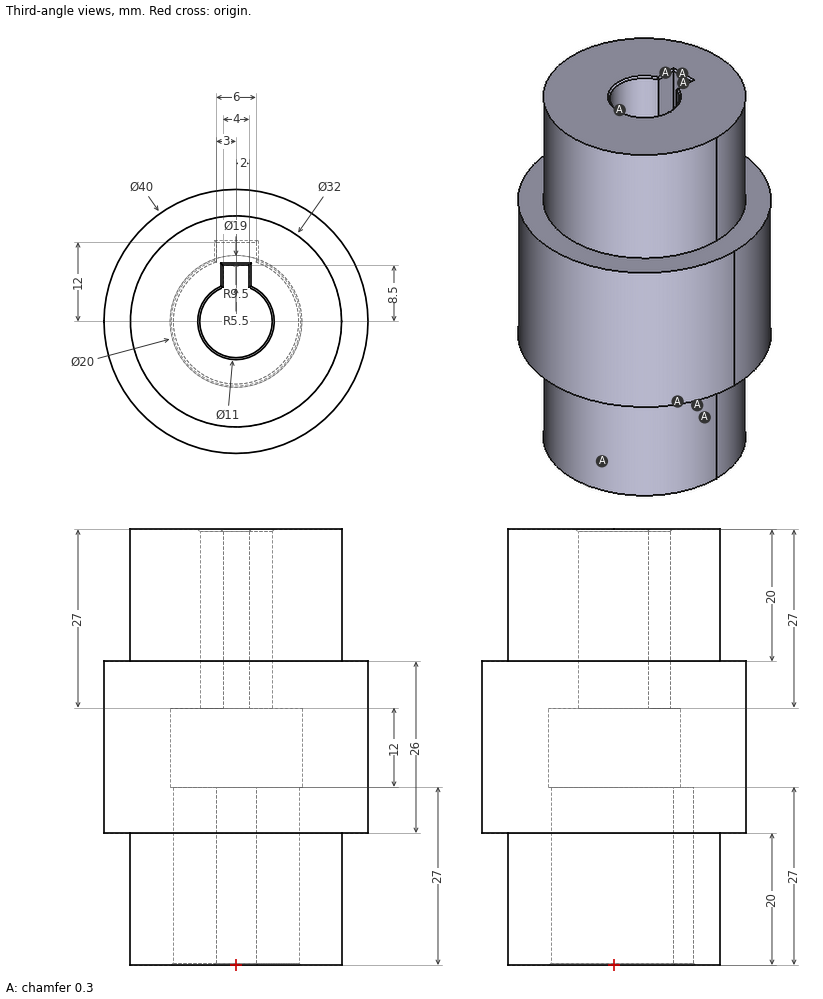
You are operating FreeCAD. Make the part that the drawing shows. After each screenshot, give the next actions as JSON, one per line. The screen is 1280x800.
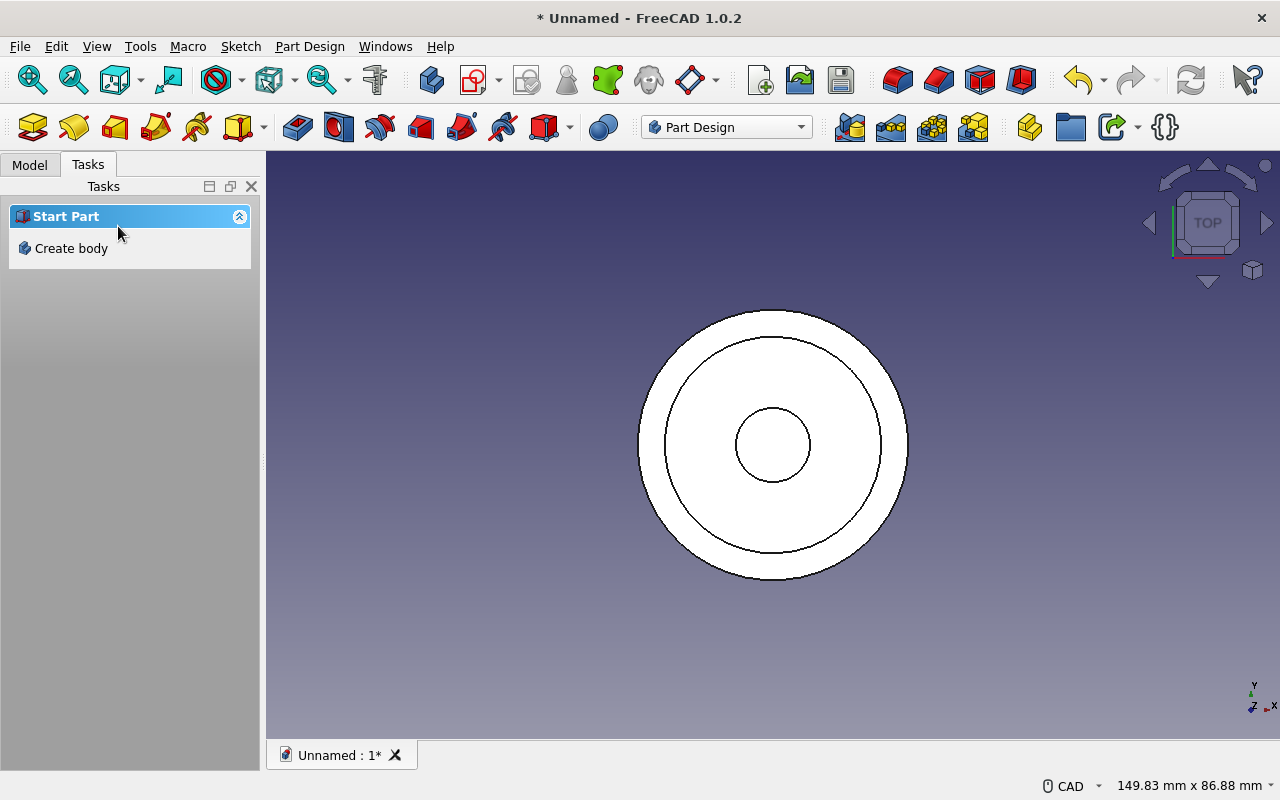
{"action": "left_click", "coordinate": [773, 444]}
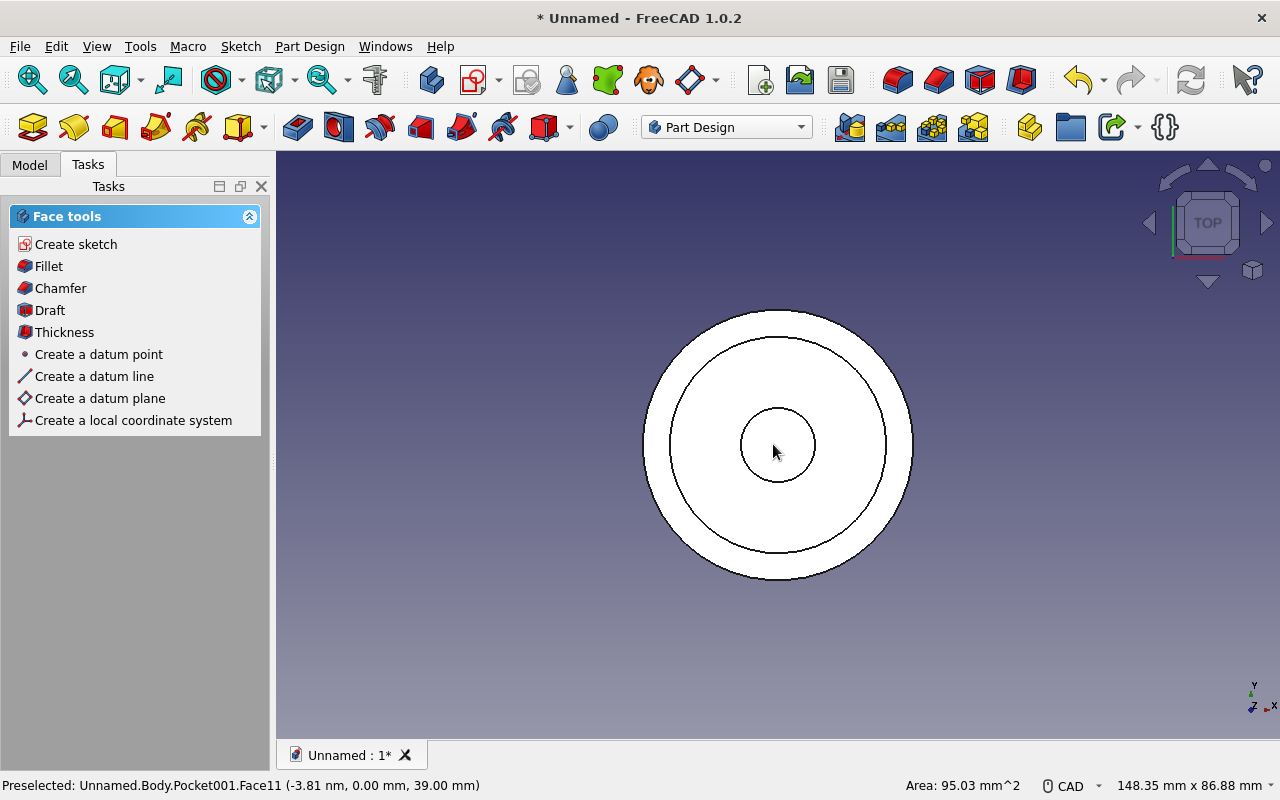
{"action": "left_click", "coordinate": [472, 80]}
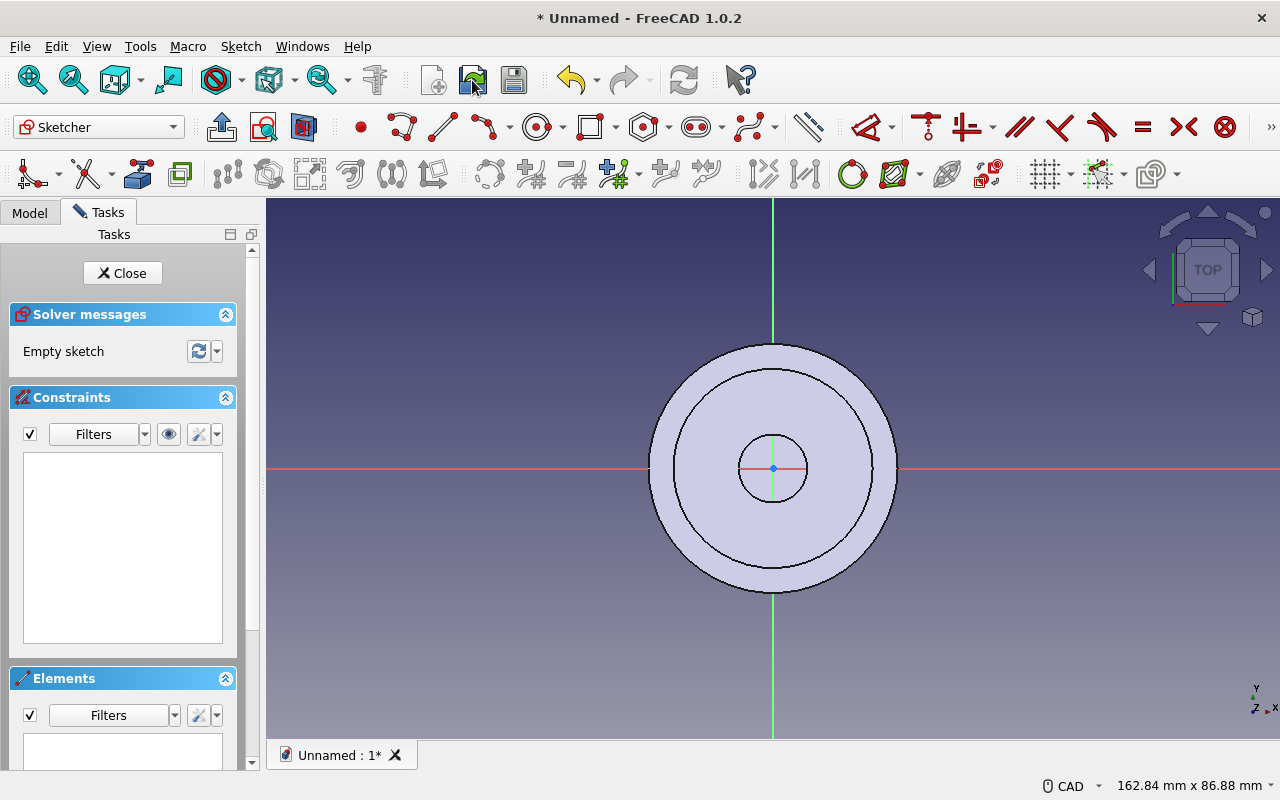
{"action": "scroll", "coordinate": [813, 468], "scroll_direction": "up", "scroll_amount": 5}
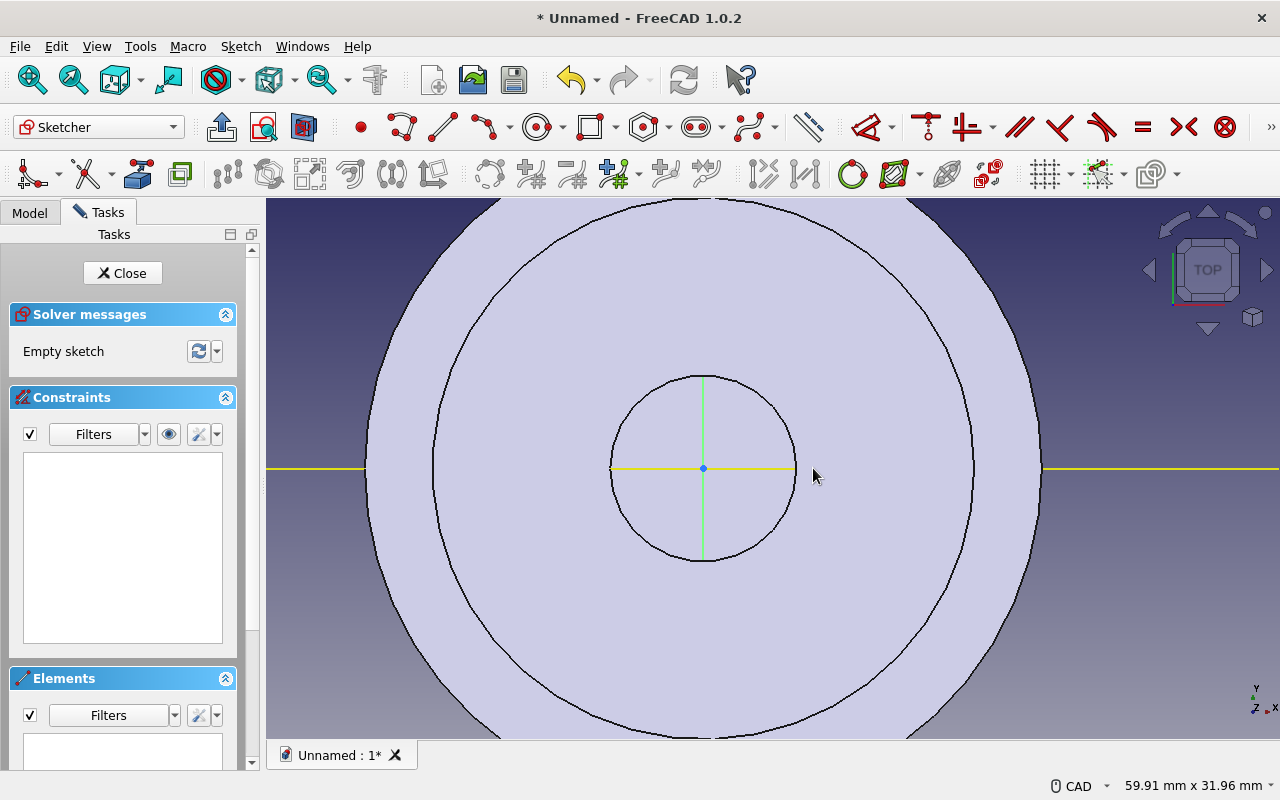
{"action": "left_click", "coordinate": [536, 128]}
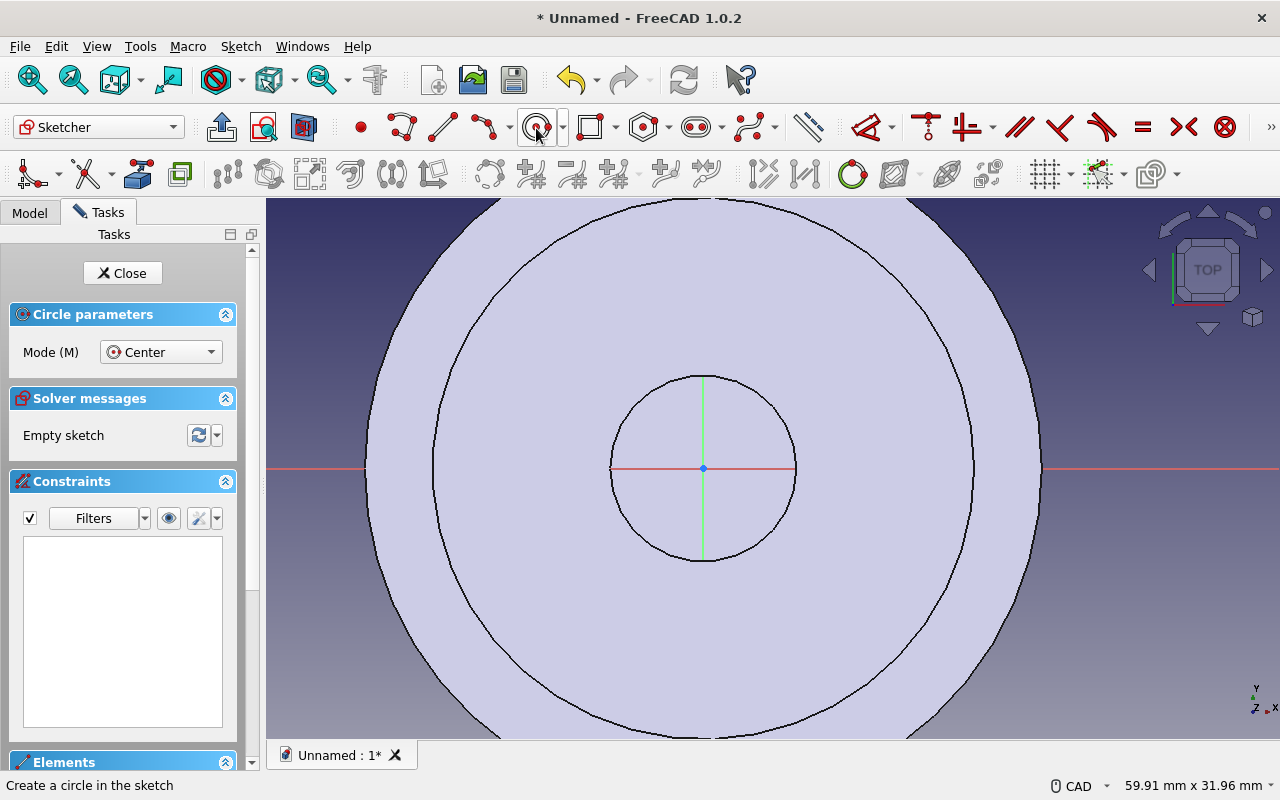
{"action": "left_click", "coordinate": [703, 468]}
{"action": "left_click", "coordinate": [823, 349]}
{"action": "key", "text": "Escape"}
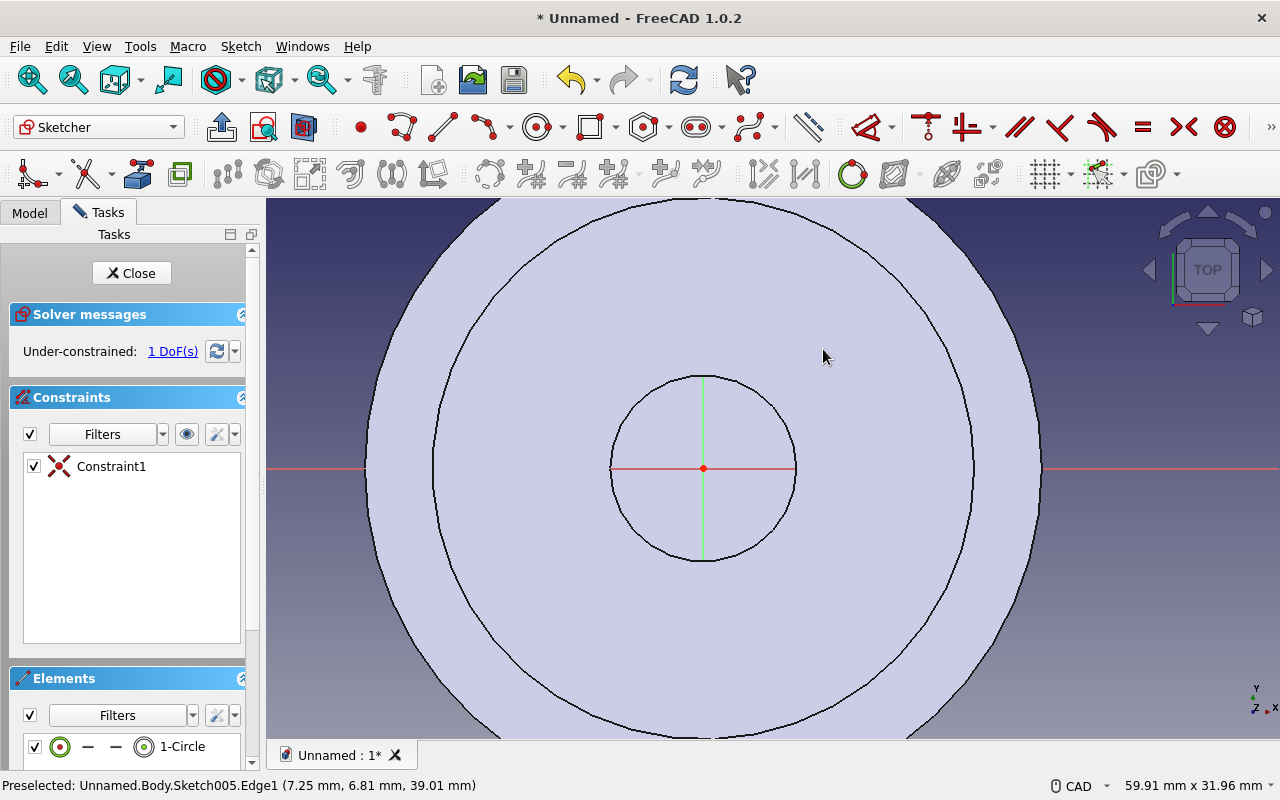
{"action": "left_click", "coordinate": [866, 128]}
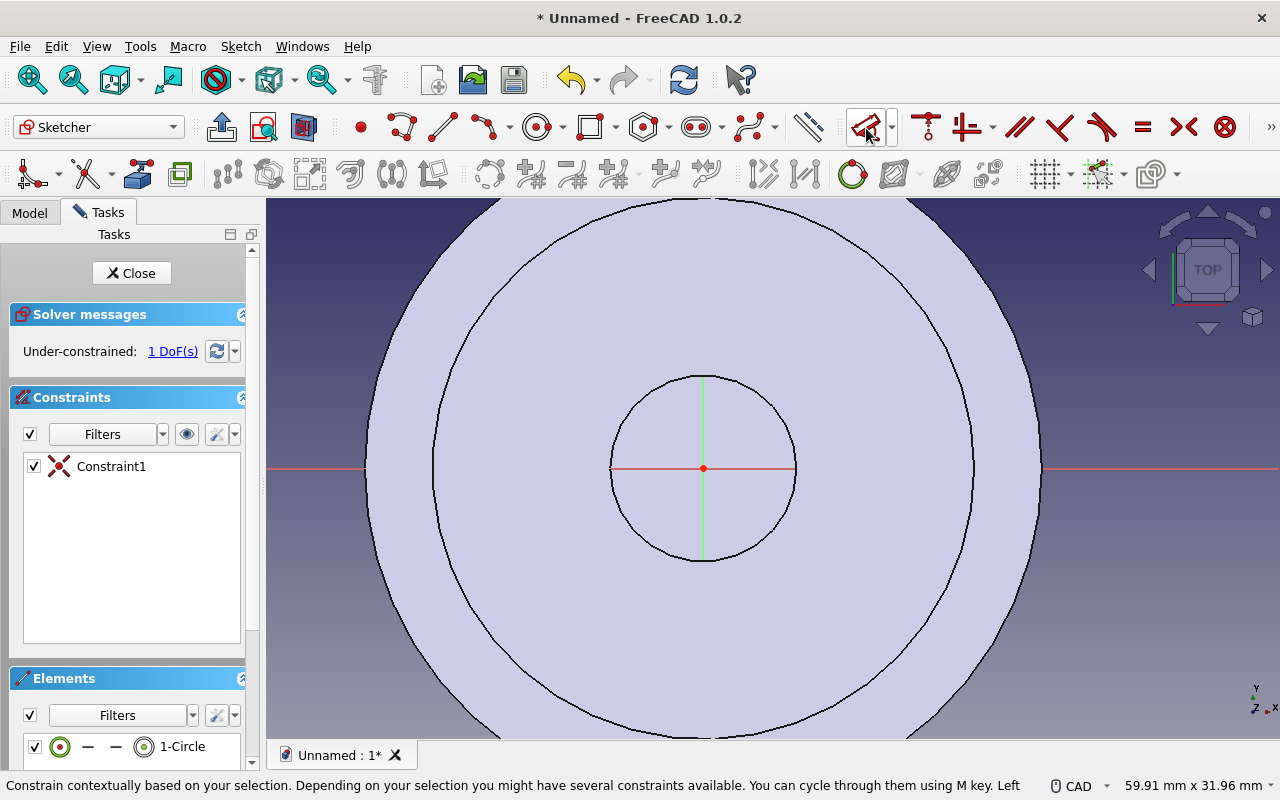
{"action": "left_click", "coordinate": [822, 349]}
{"action": "left_click", "coordinate": [845, 326]}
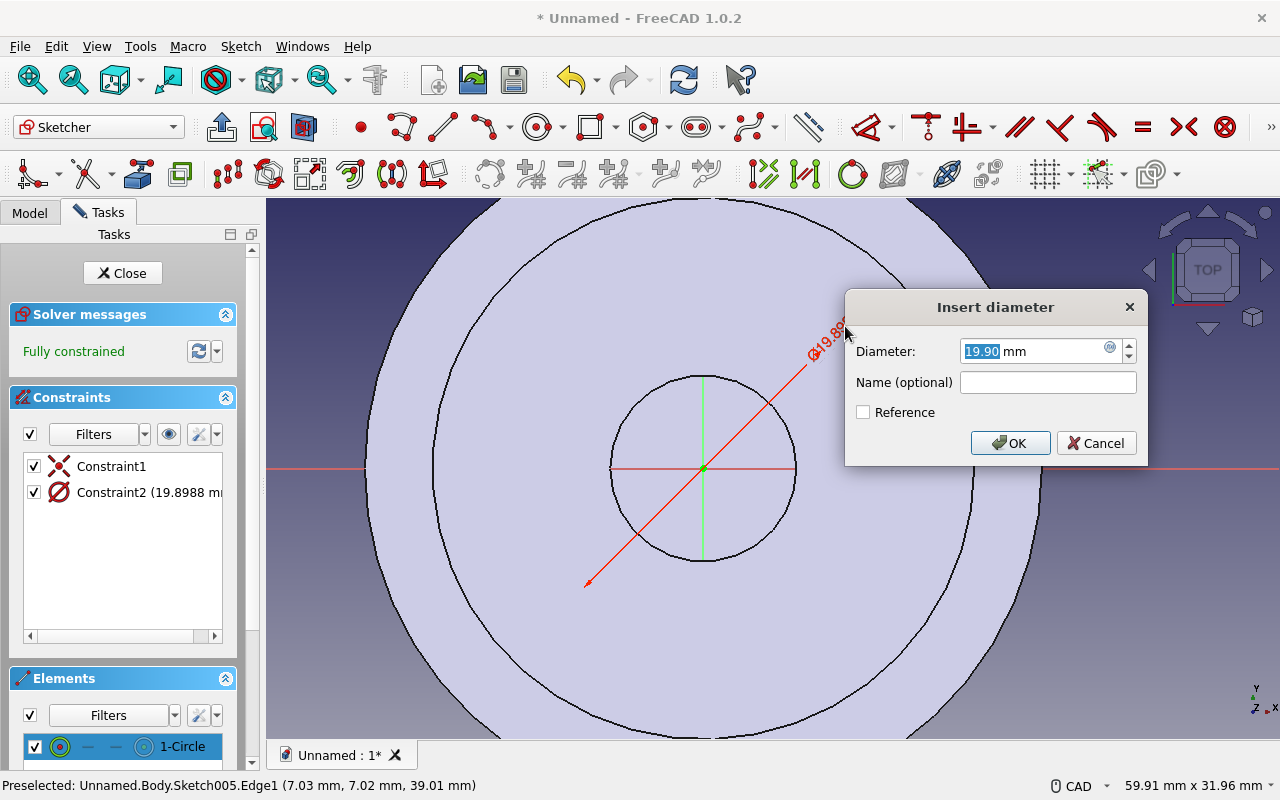
{"action": "type", "text": "20"}
{"action": "key", "text": "Return"}
{"action": "key", "text": "Escape"}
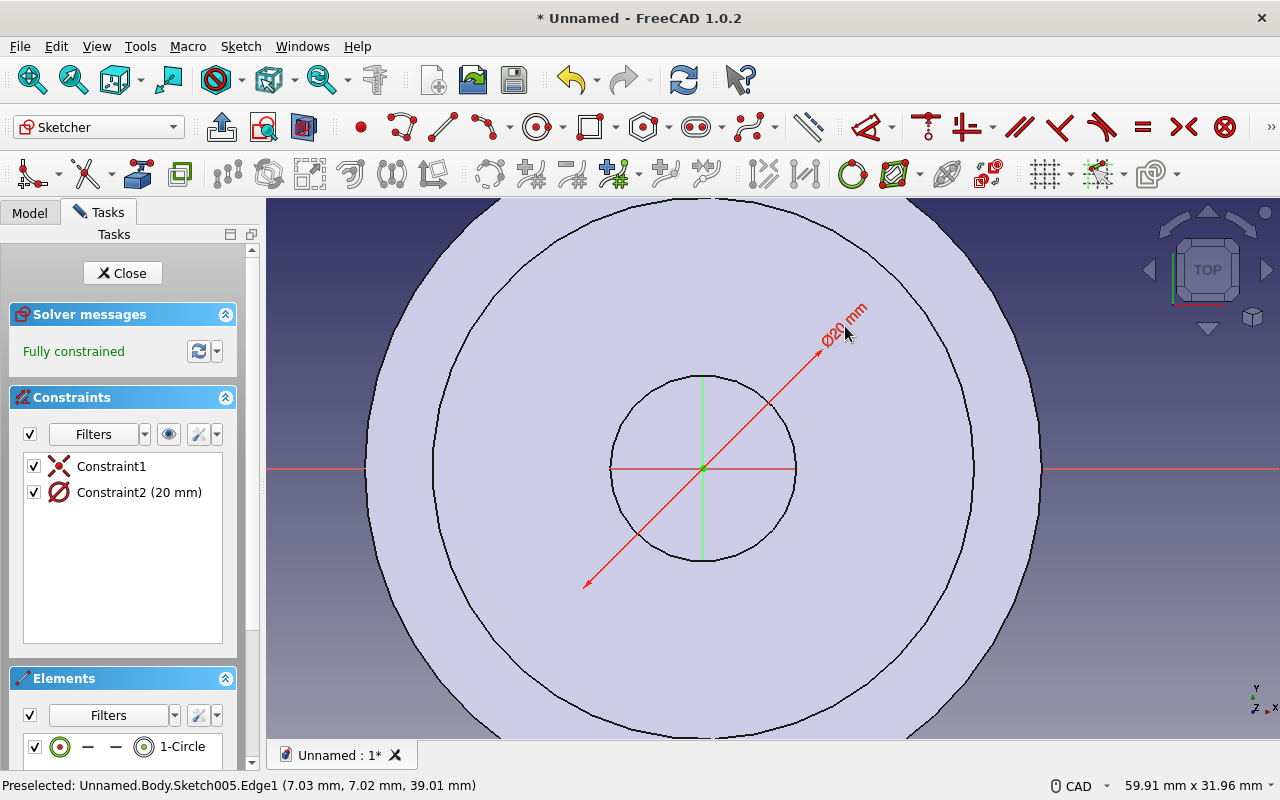
{"action": "left_click", "coordinate": [123, 273]}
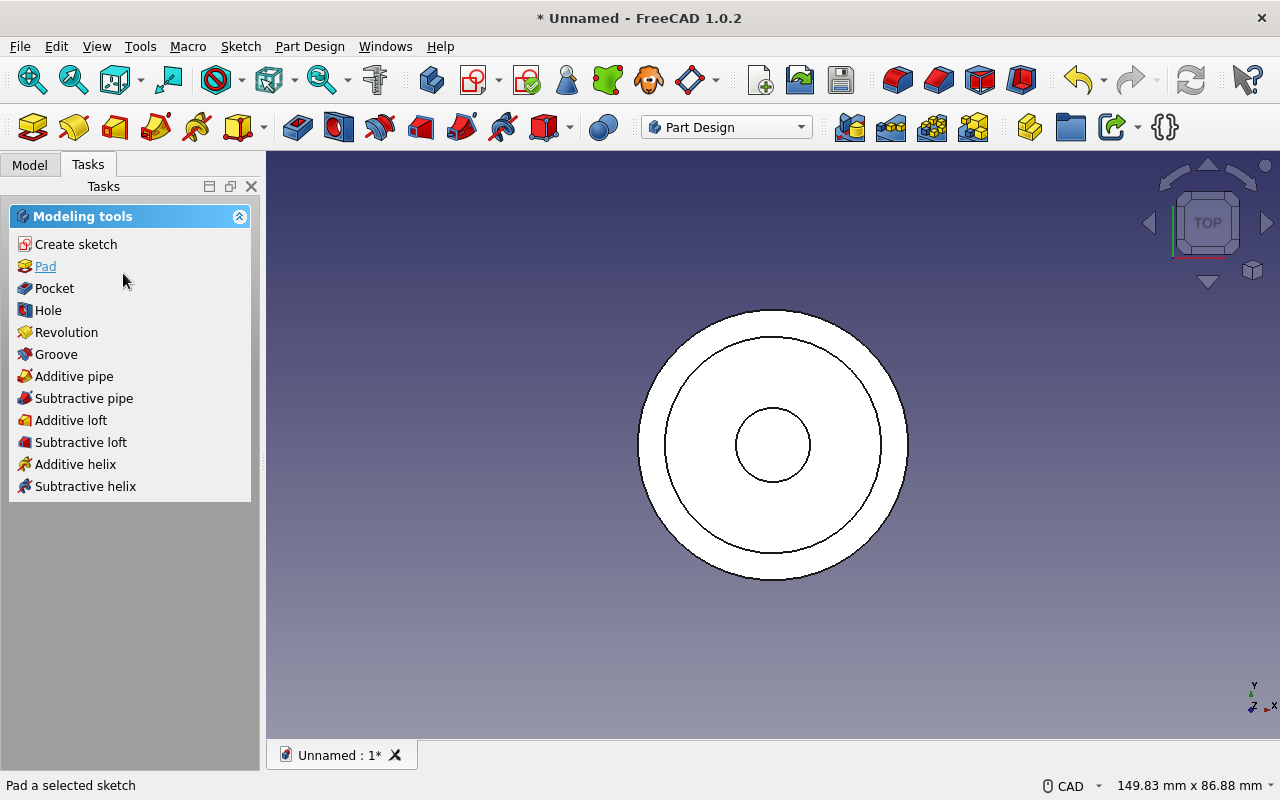
{"action": "left_click", "coordinate": [298, 128]}